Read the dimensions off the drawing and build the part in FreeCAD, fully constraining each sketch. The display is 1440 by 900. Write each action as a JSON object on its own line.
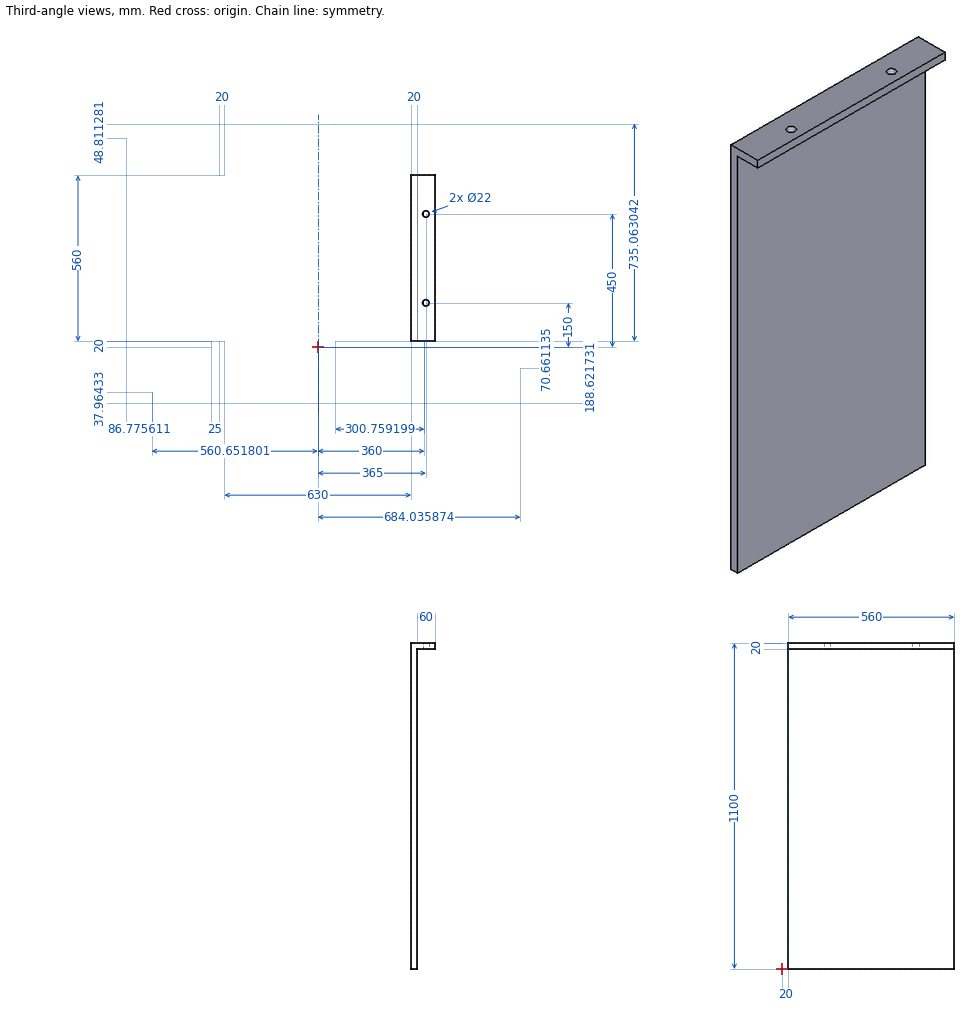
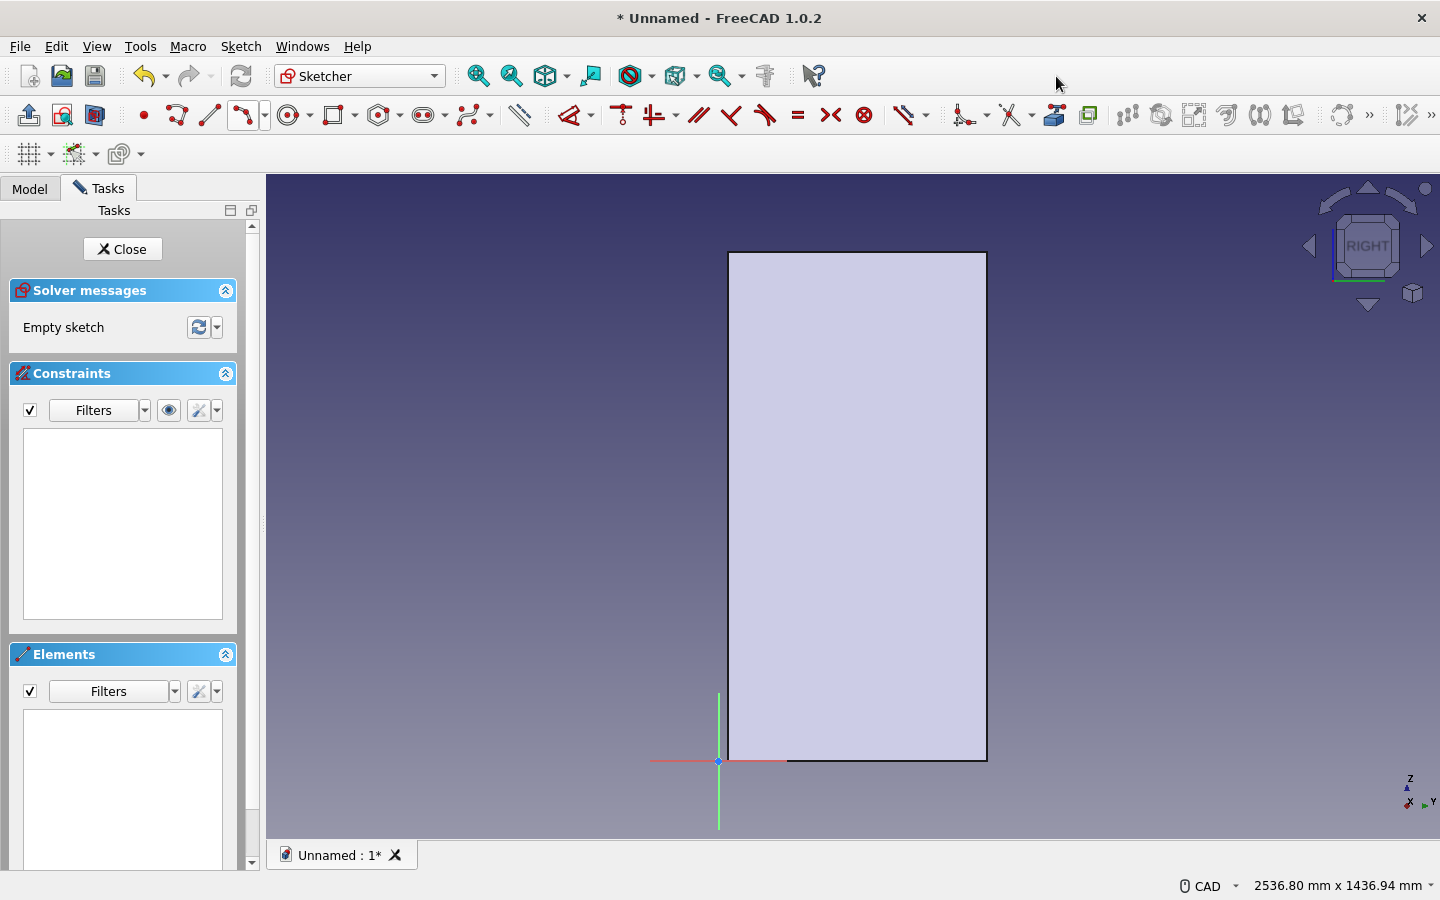
{"action": "left_click", "coordinate": [332, 116]}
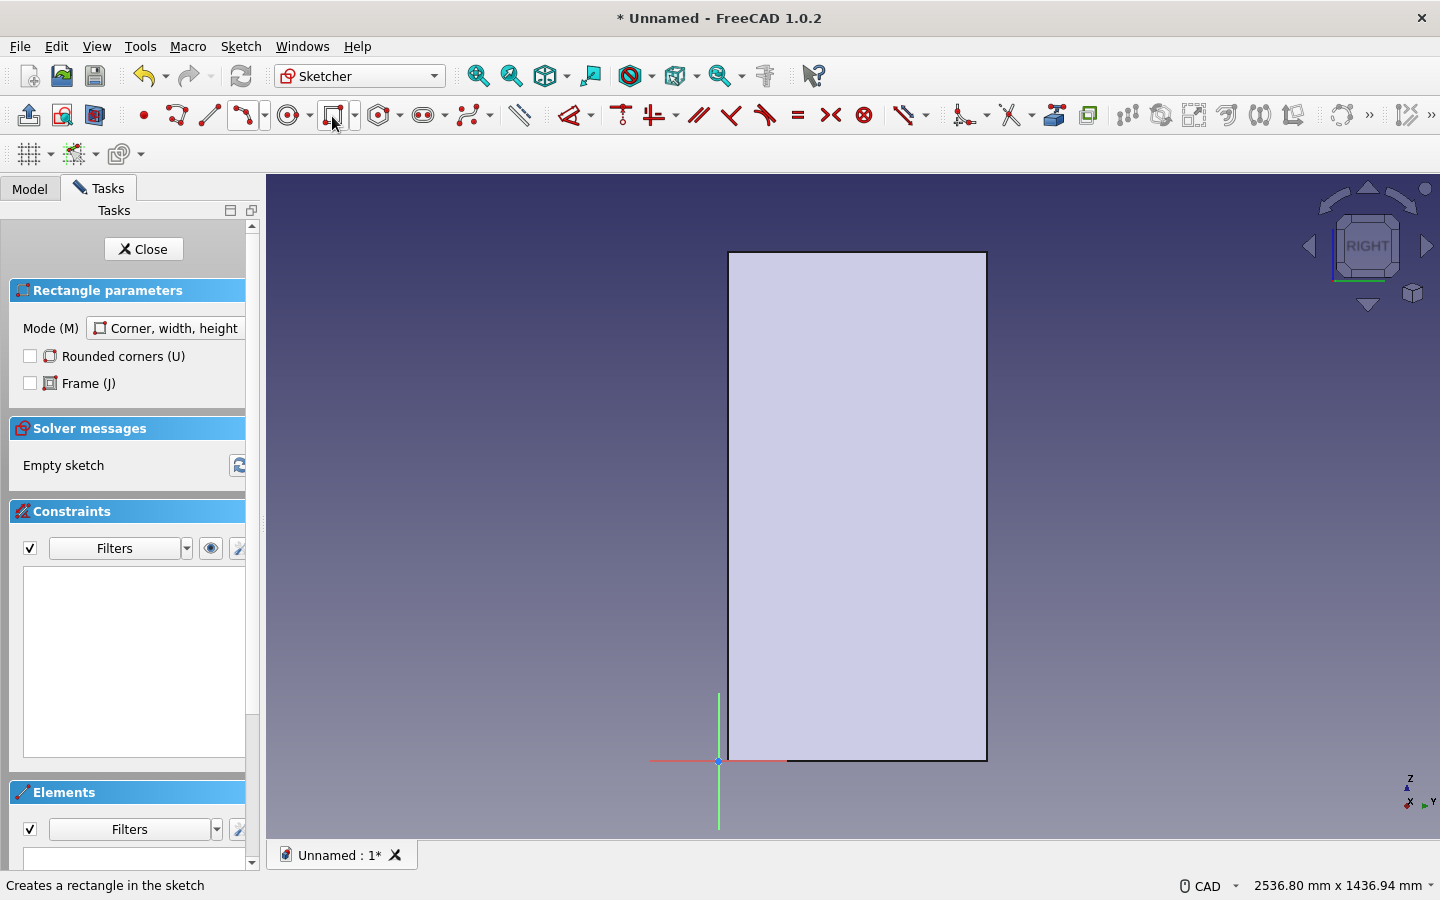
{"action": "scroll", "coordinate": [728, 252], "scroll_direction": "up", "scroll_amount": 3}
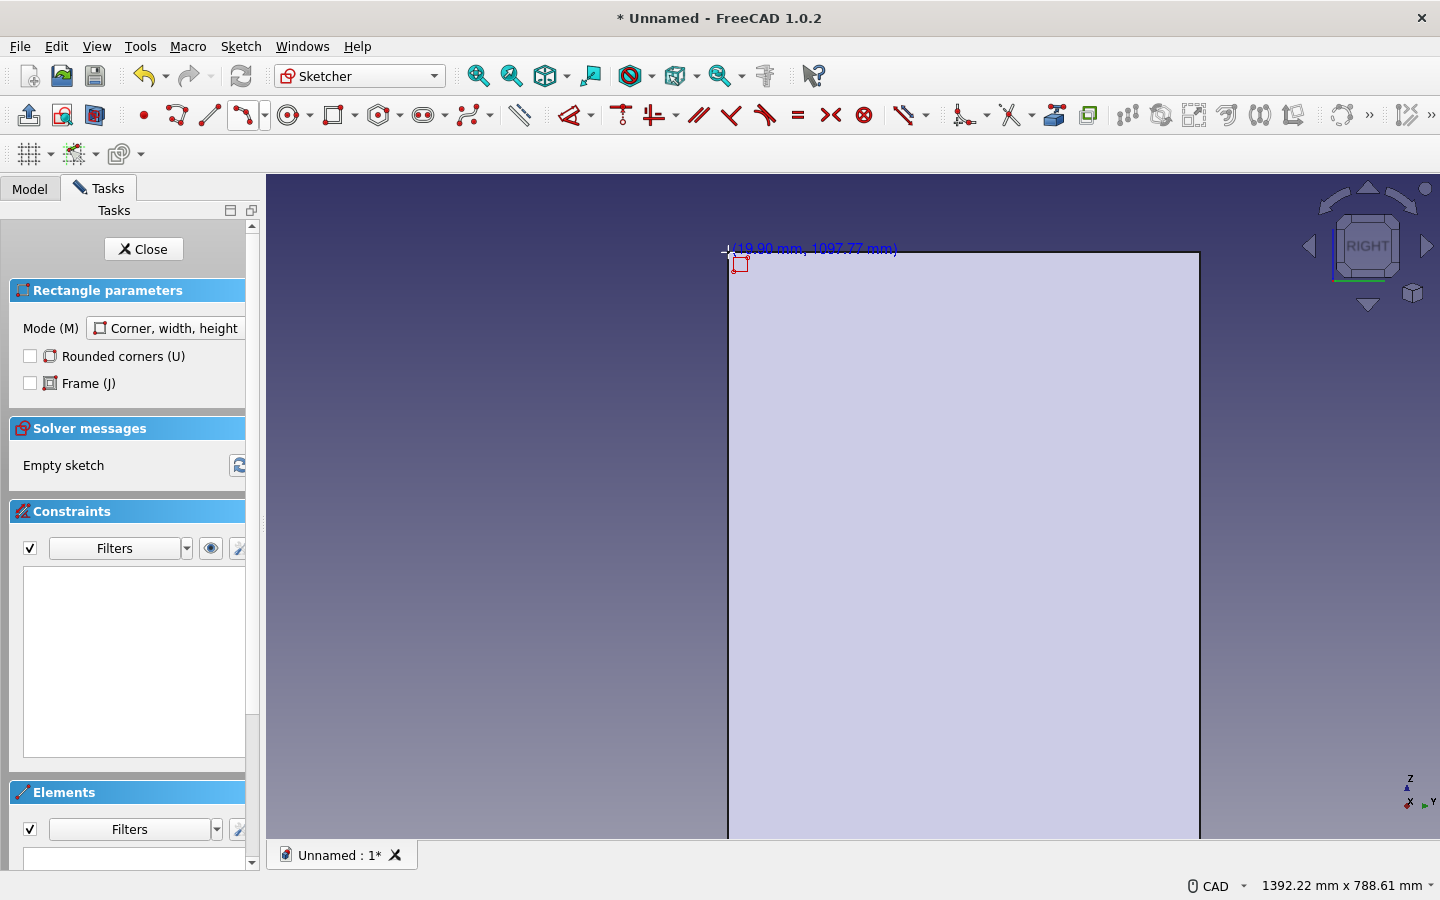
{"action": "left_click", "coordinate": [728, 252]}
{"action": "left_click", "coordinate": [1200, 269]}
{"action": "key", "text": "Escape"}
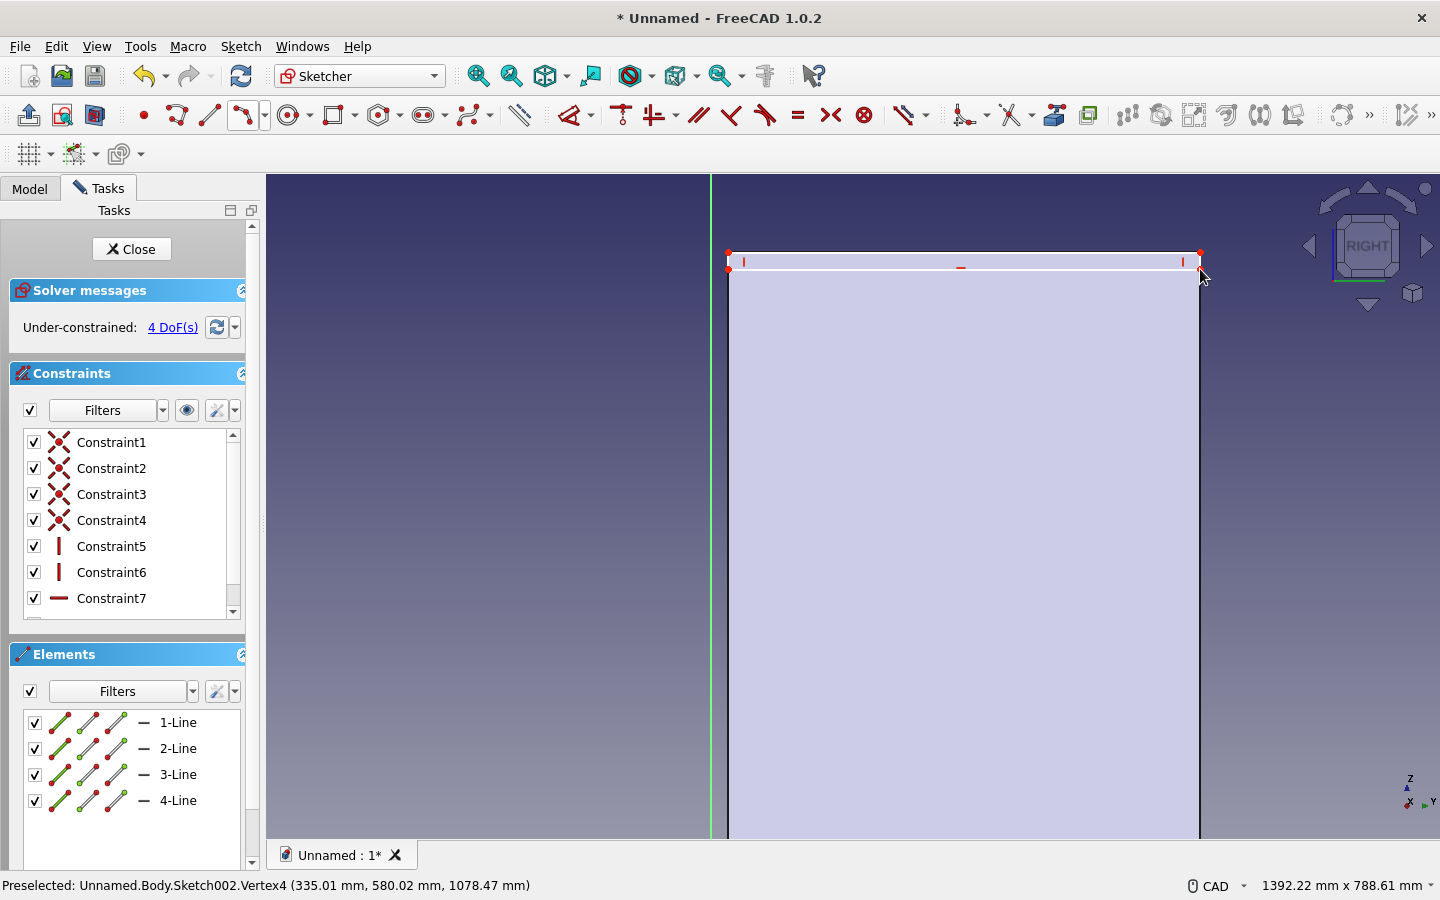
{"action": "left_click", "coordinate": [568, 116]}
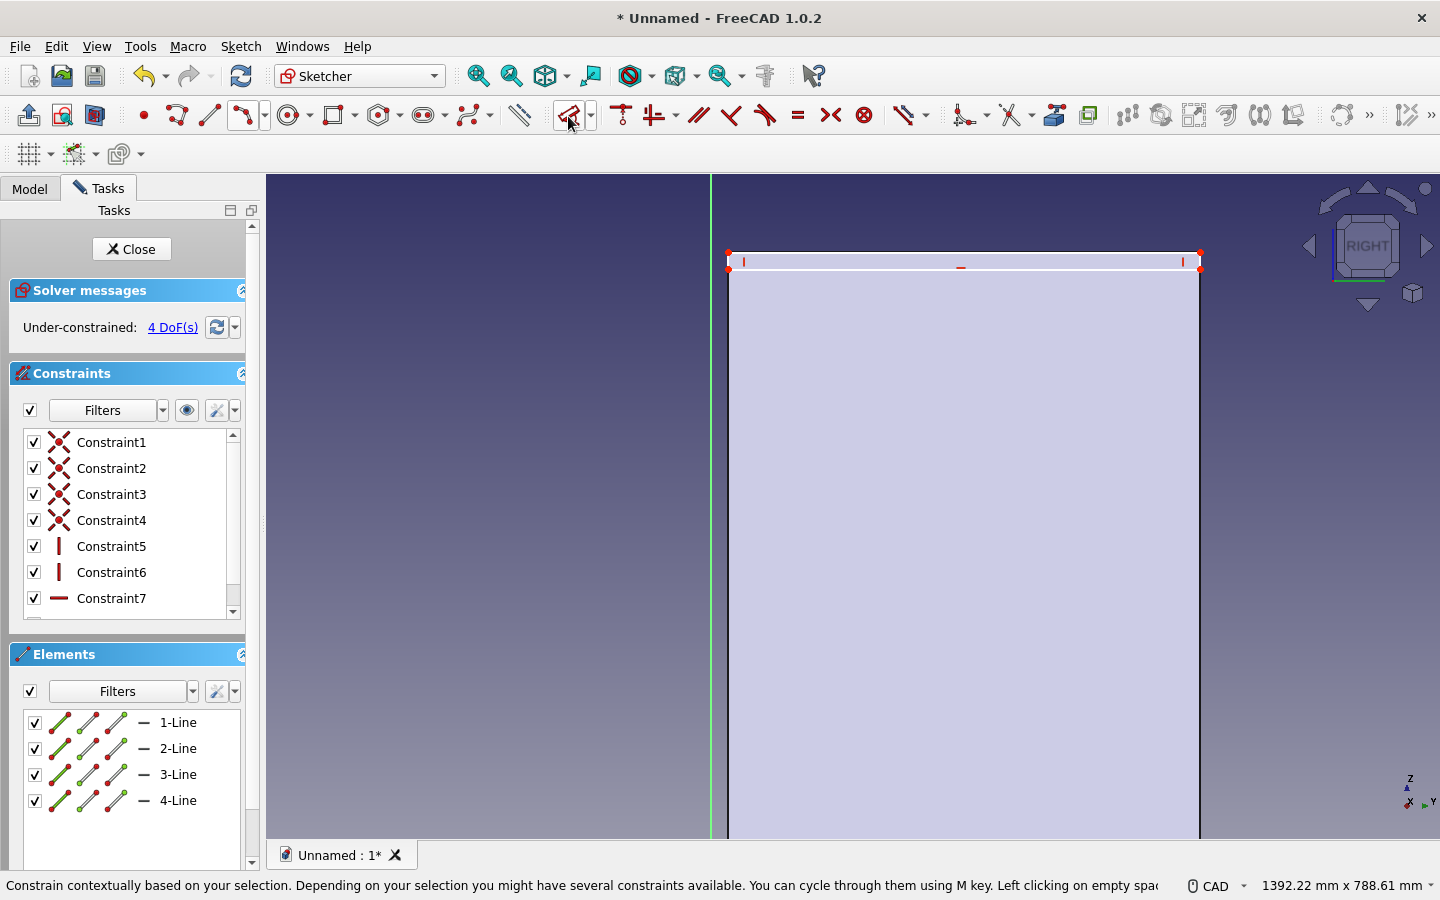
{"action": "scroll", "coordinate": [728, 262], "scroll_direction": "up", "scroll_amount": 5}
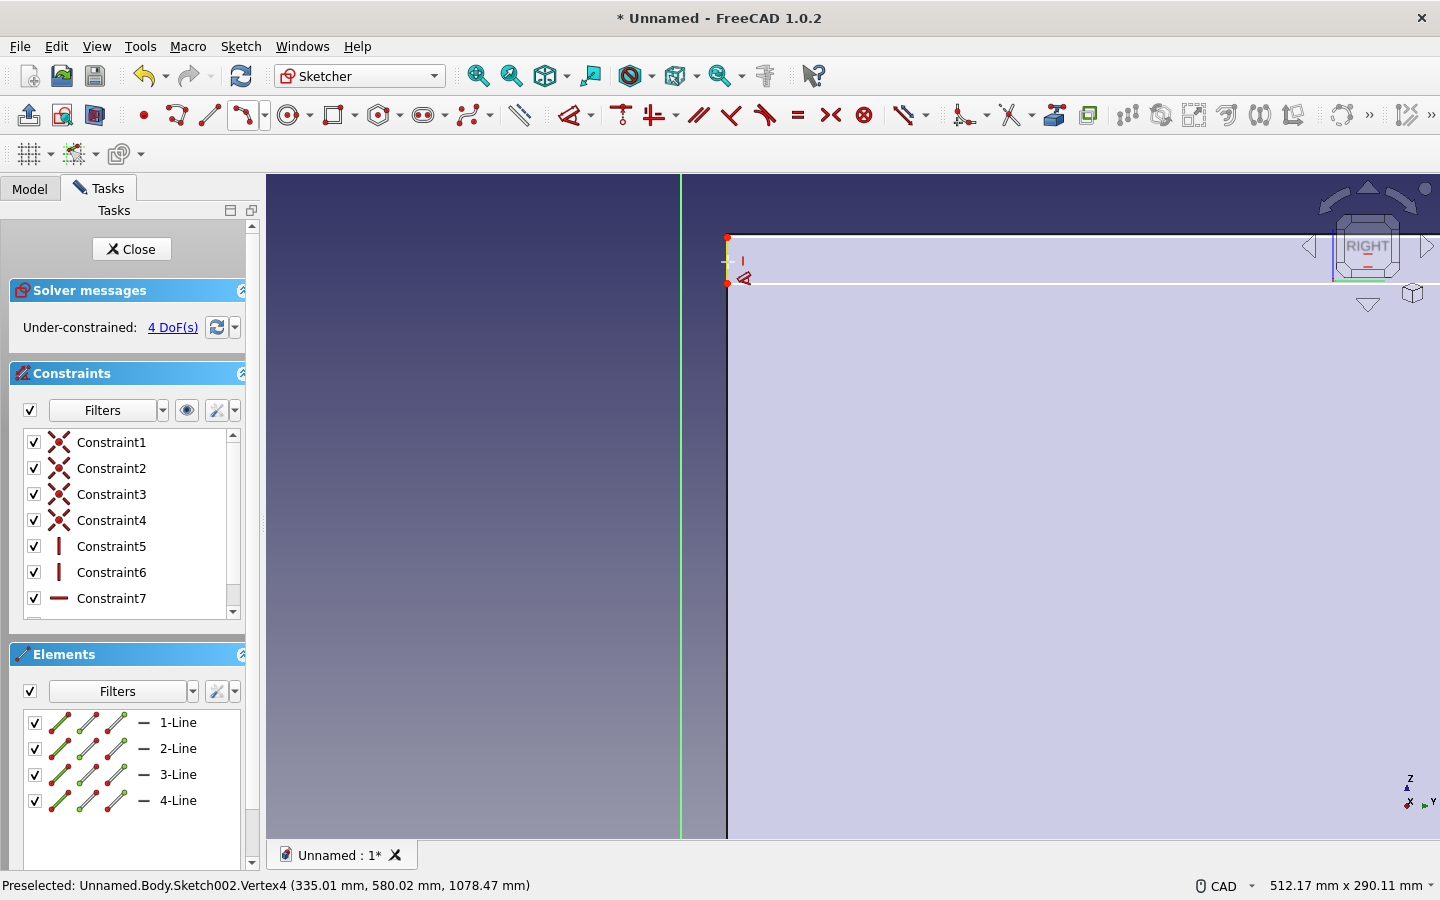
{"action": "left_click", "coordinate": [727, 260]}
{"action": "left_click", "coordinate": [761, 260]}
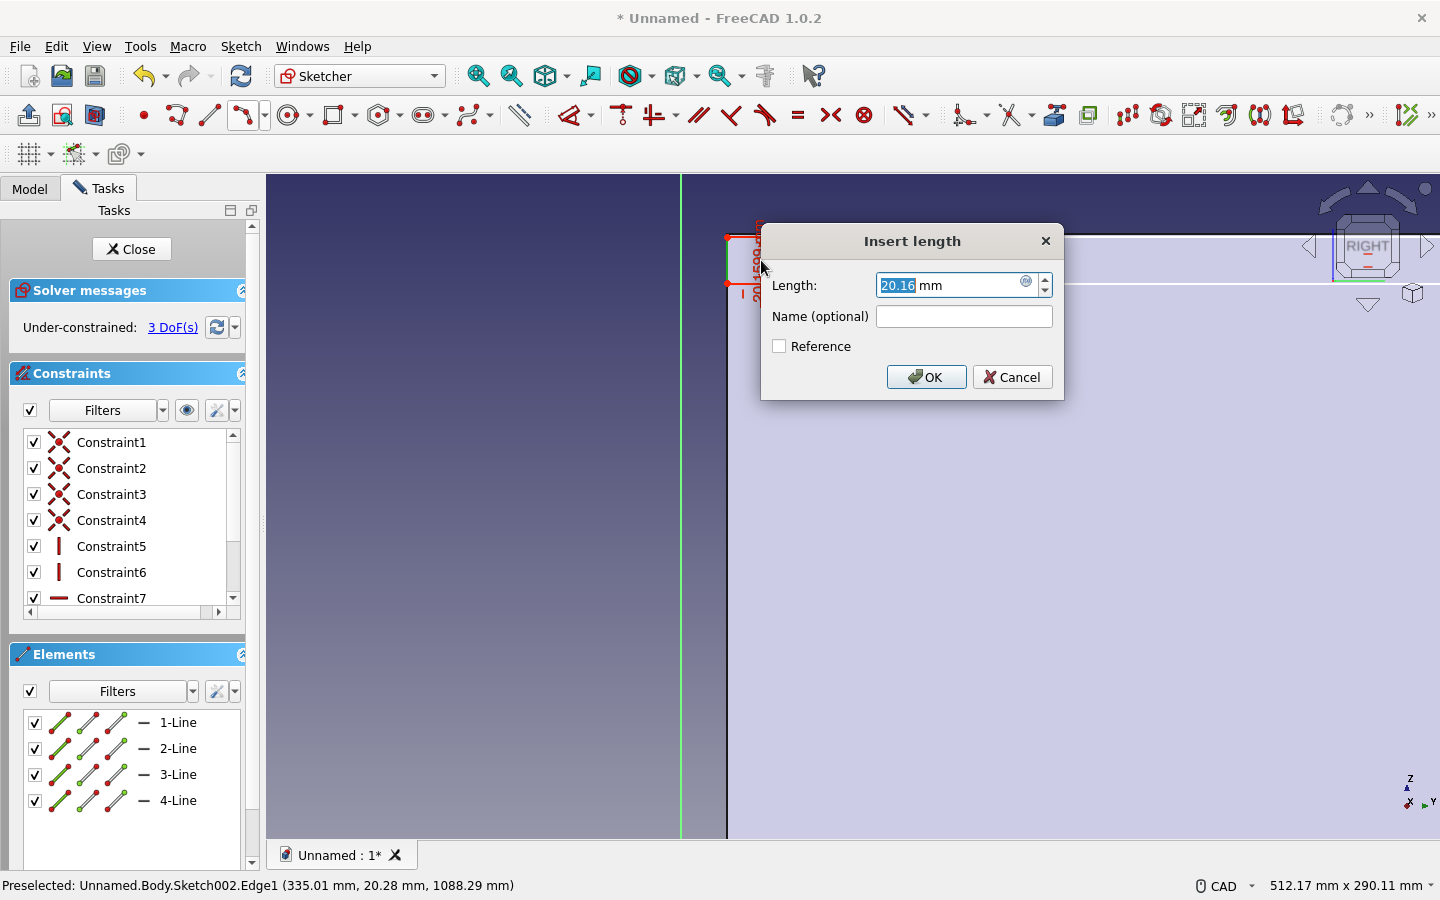
{"action": "type", "text": "20"}
{"action": "key", "text": "Return"}